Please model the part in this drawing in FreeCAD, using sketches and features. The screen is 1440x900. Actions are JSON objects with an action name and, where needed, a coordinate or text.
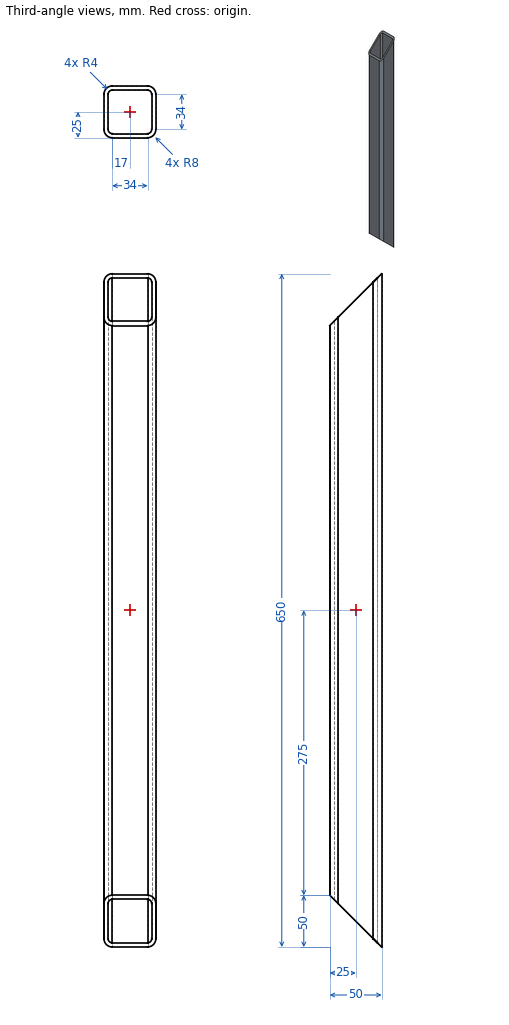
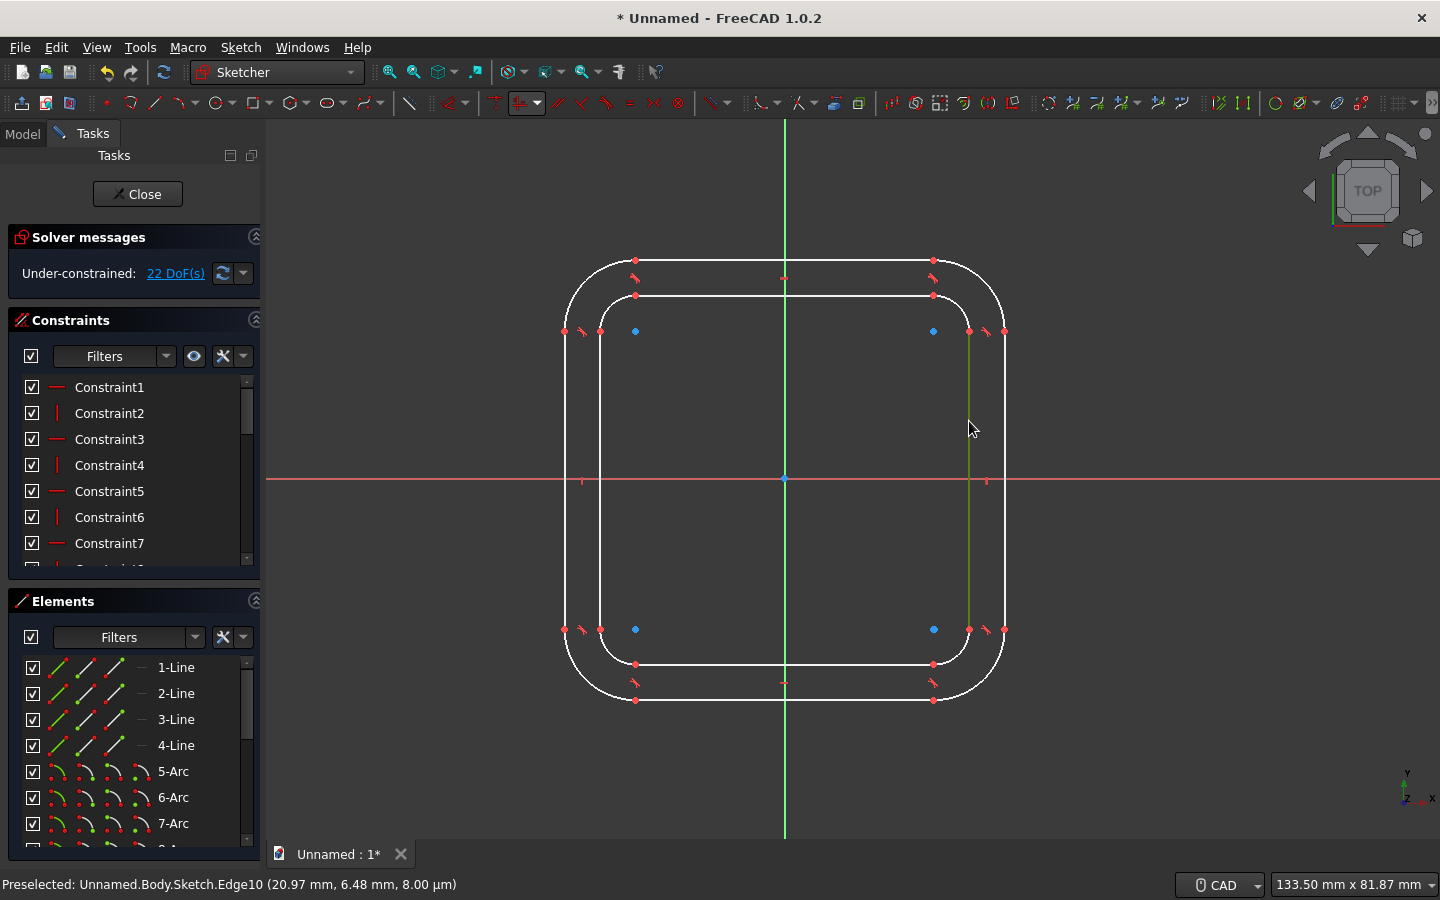
{"action": "left_click", "coordinate": [965, 315]}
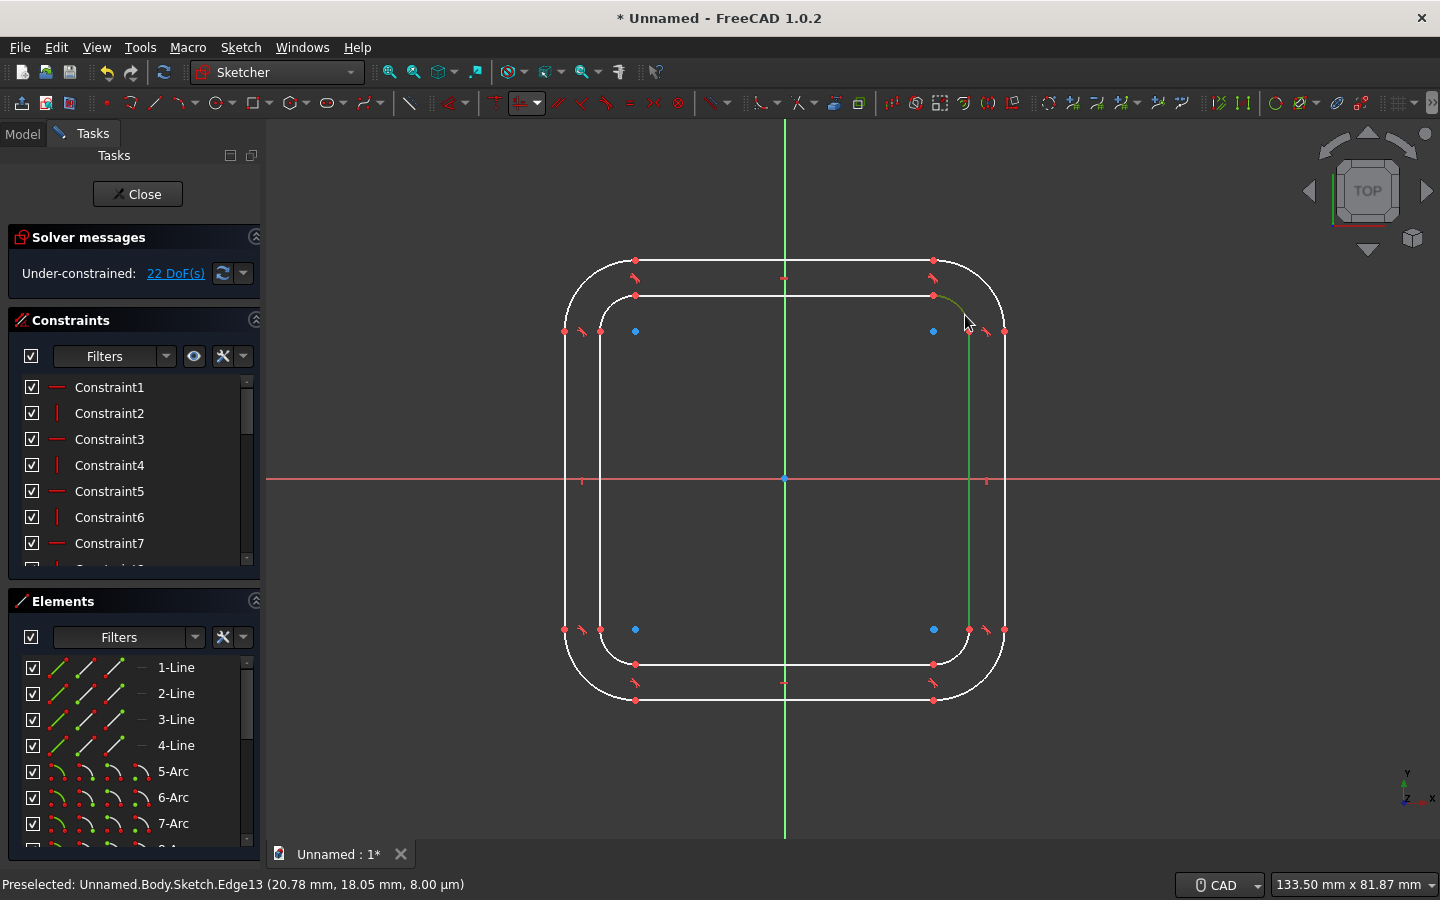
{"action": "left_click", "coordinate": [606, 104]}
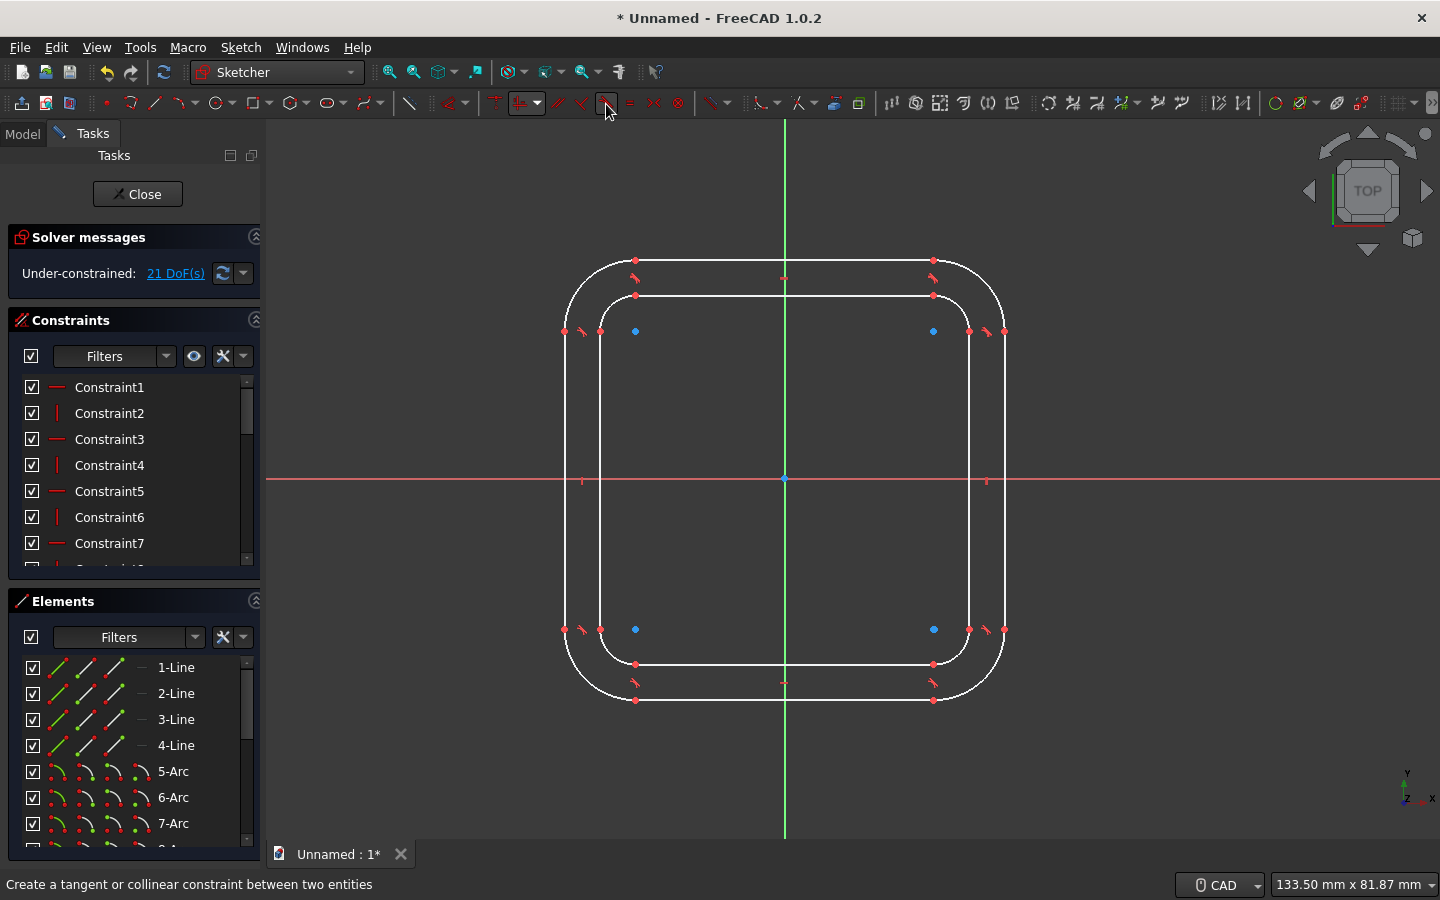
{"action": "left_click", "coordinate": [969, 421]}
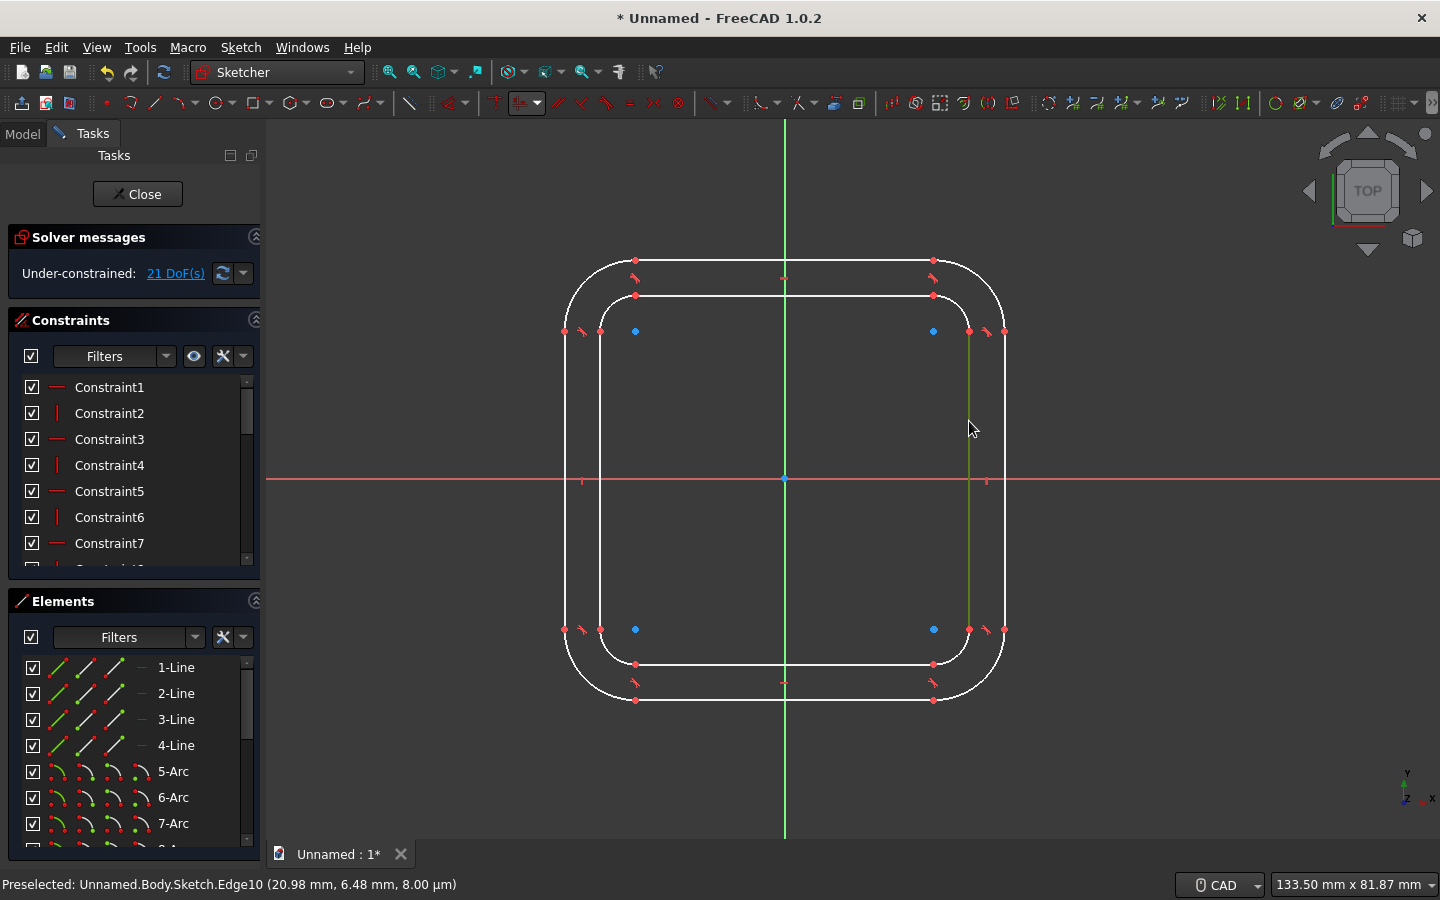
{"action": "left_click", "coordinate": [950, 661]}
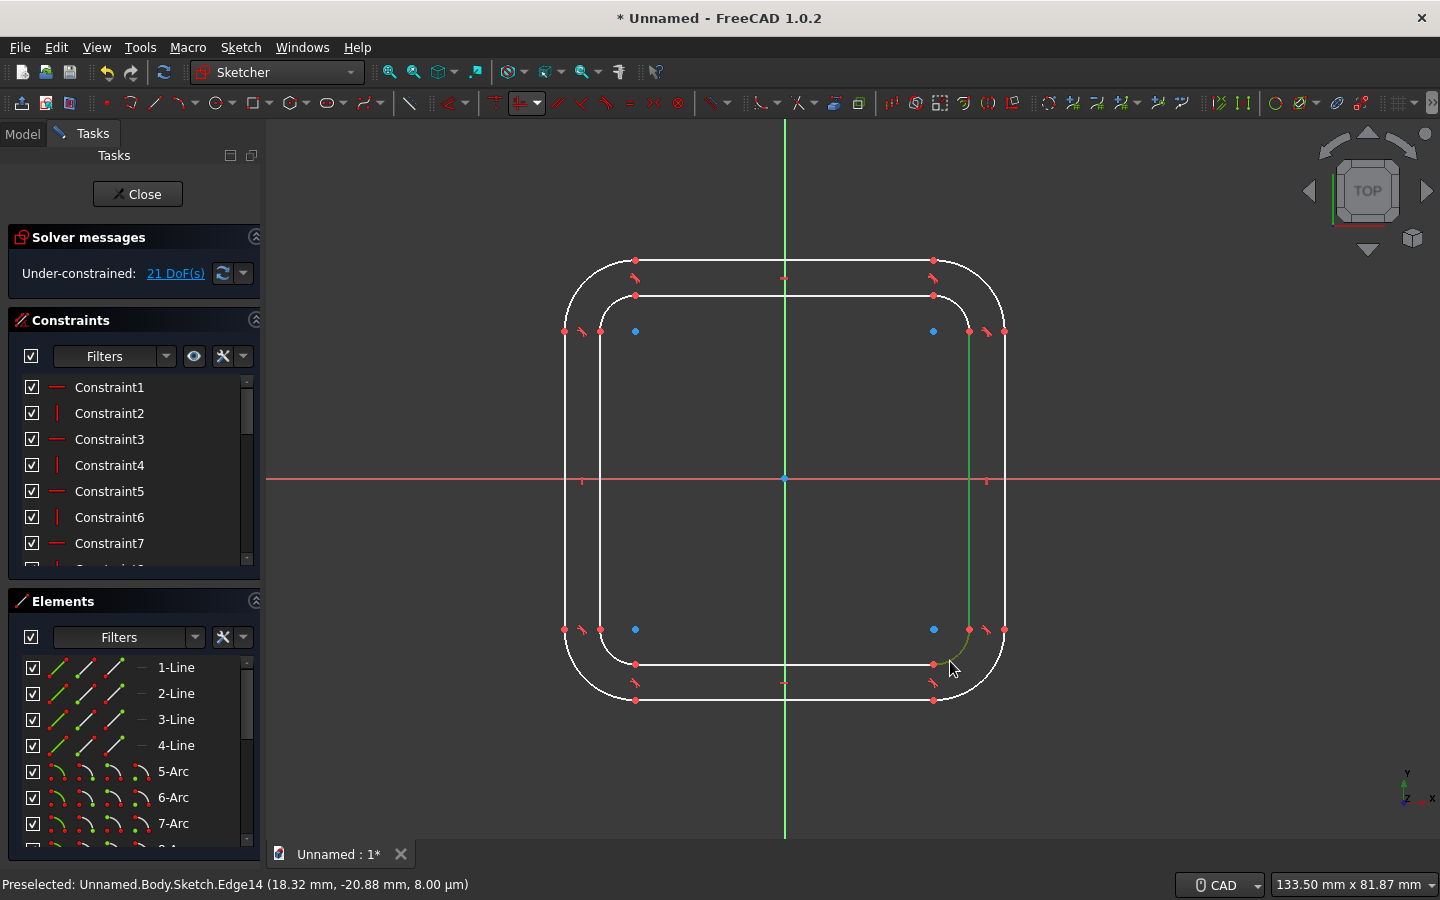
{"action": "left_click", "coordinate": [606, 104]}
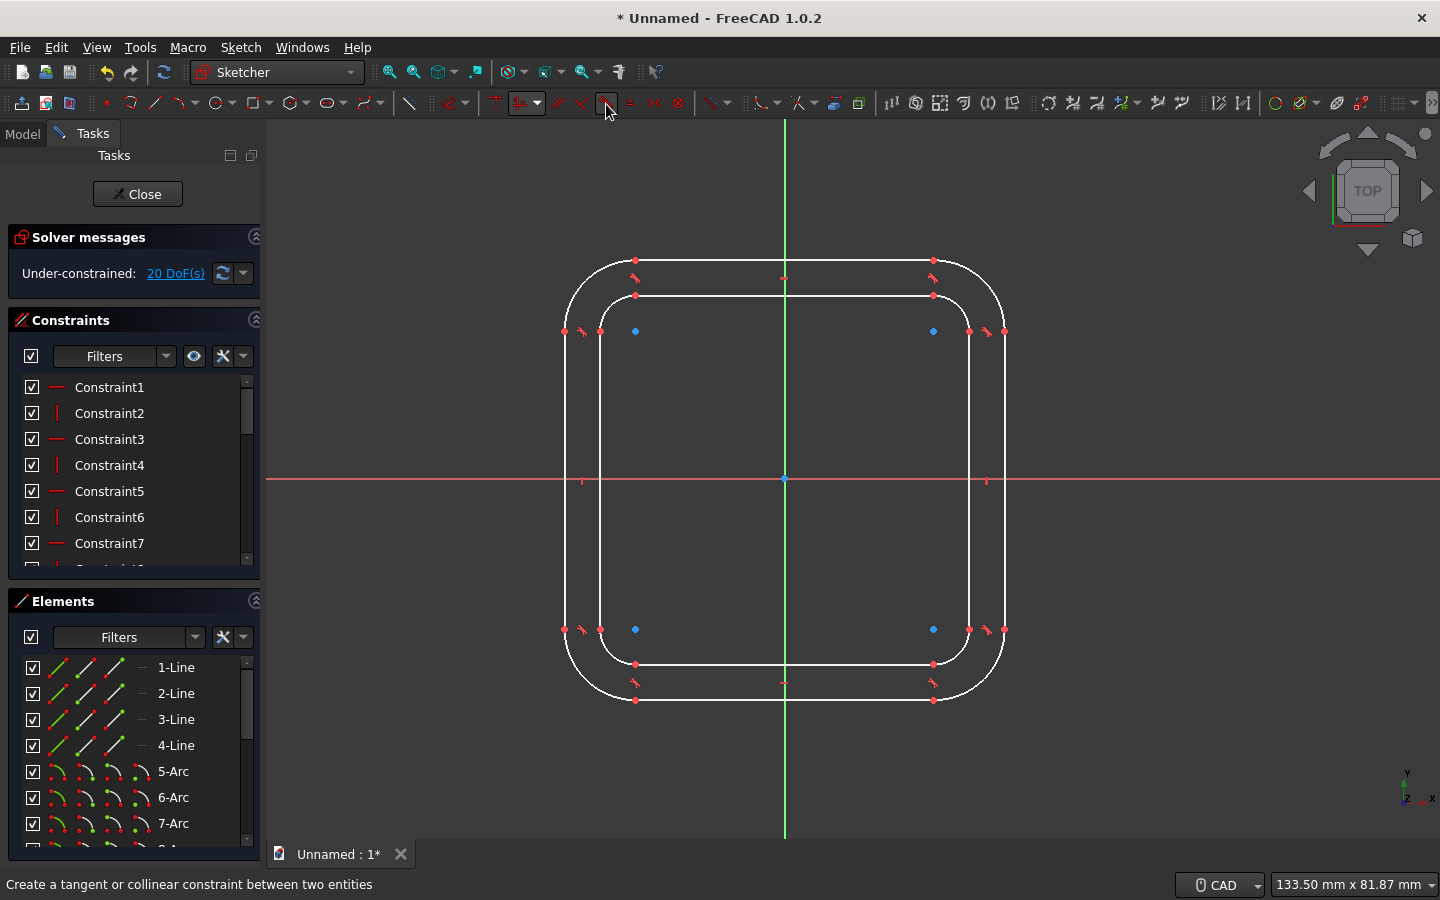
{"action": "left_click", "coordinate": [844, 665]}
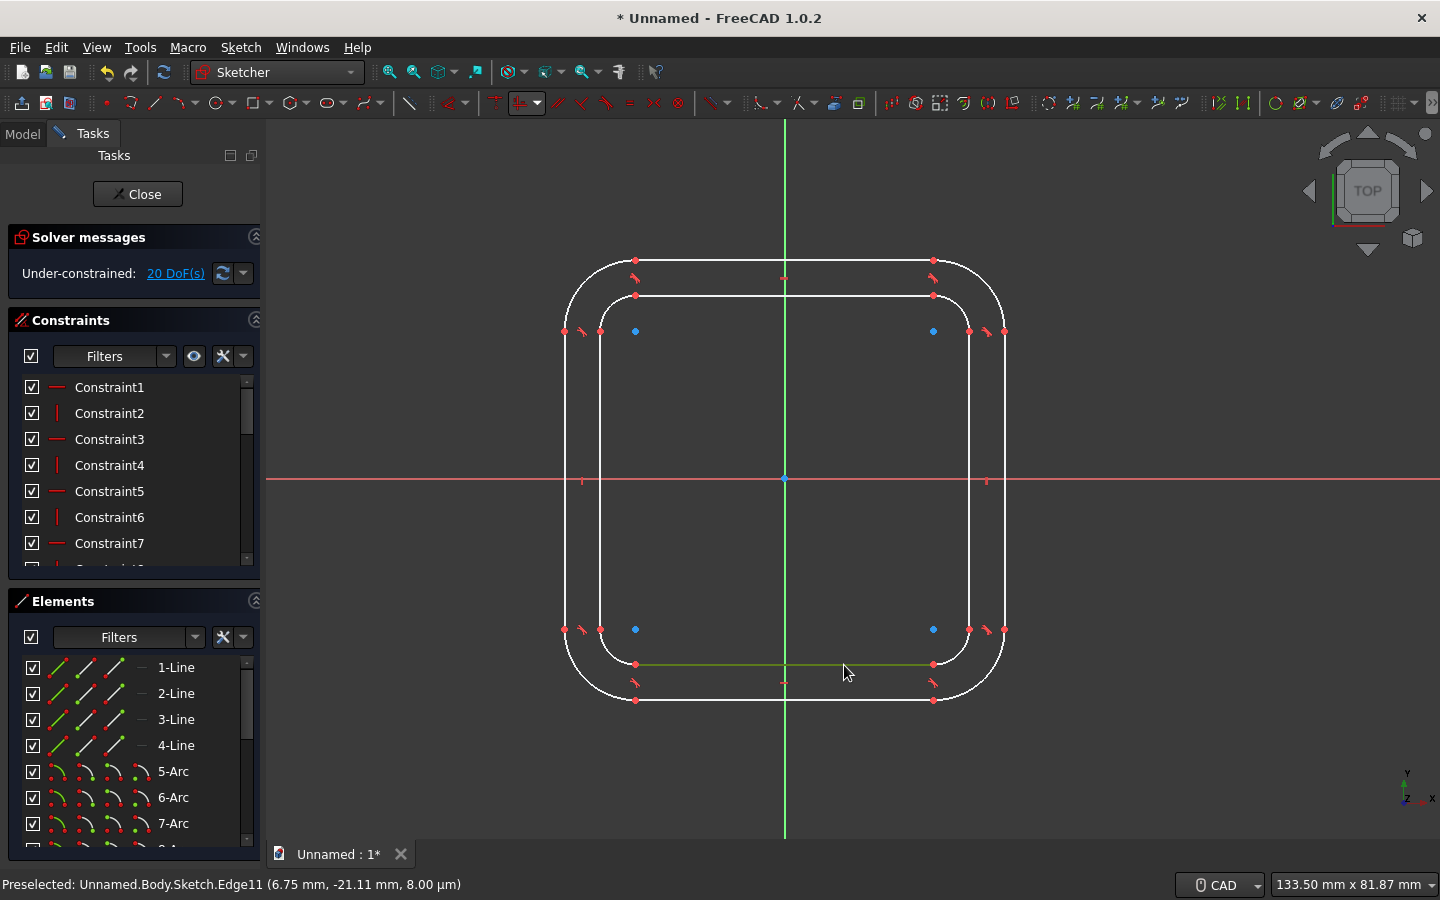
{"action": "left_click", "coordinate": [950, 661]}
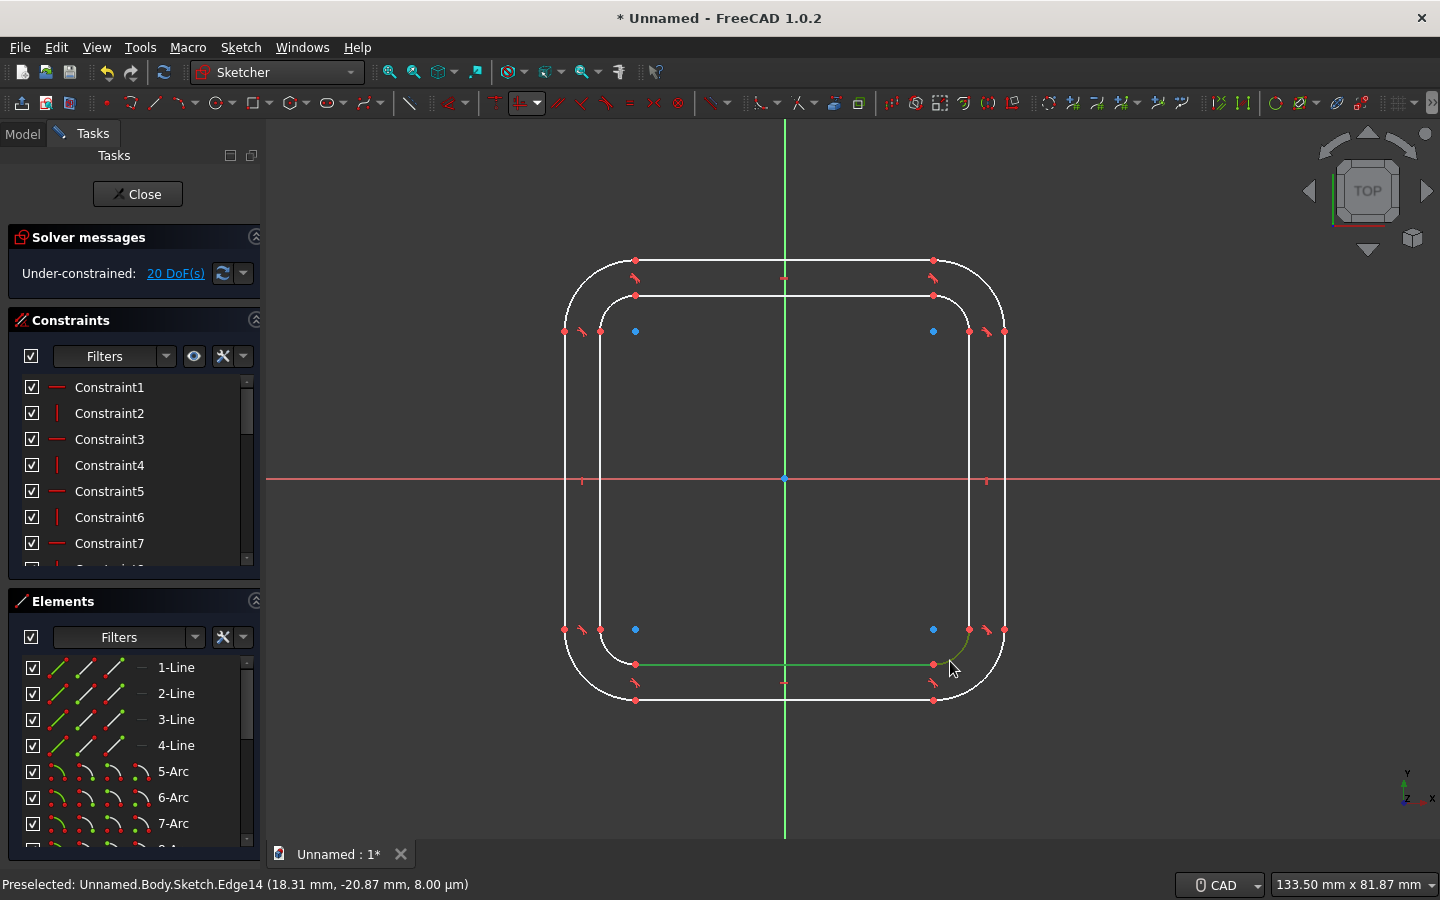
{"action": "key", "text": "t"}